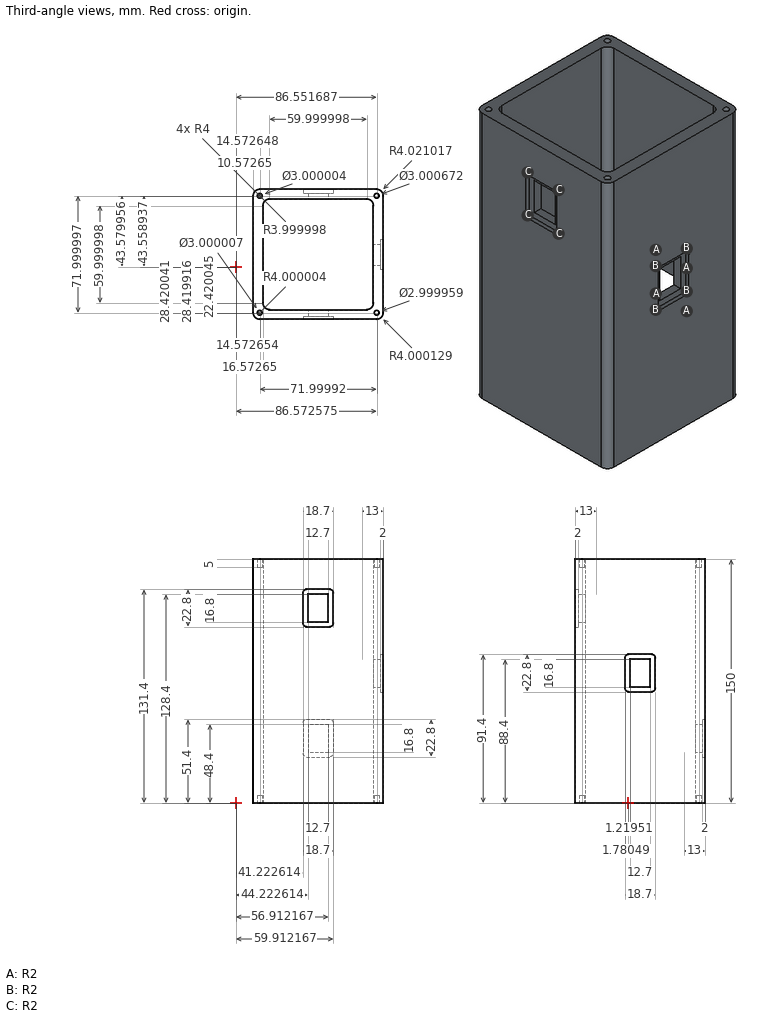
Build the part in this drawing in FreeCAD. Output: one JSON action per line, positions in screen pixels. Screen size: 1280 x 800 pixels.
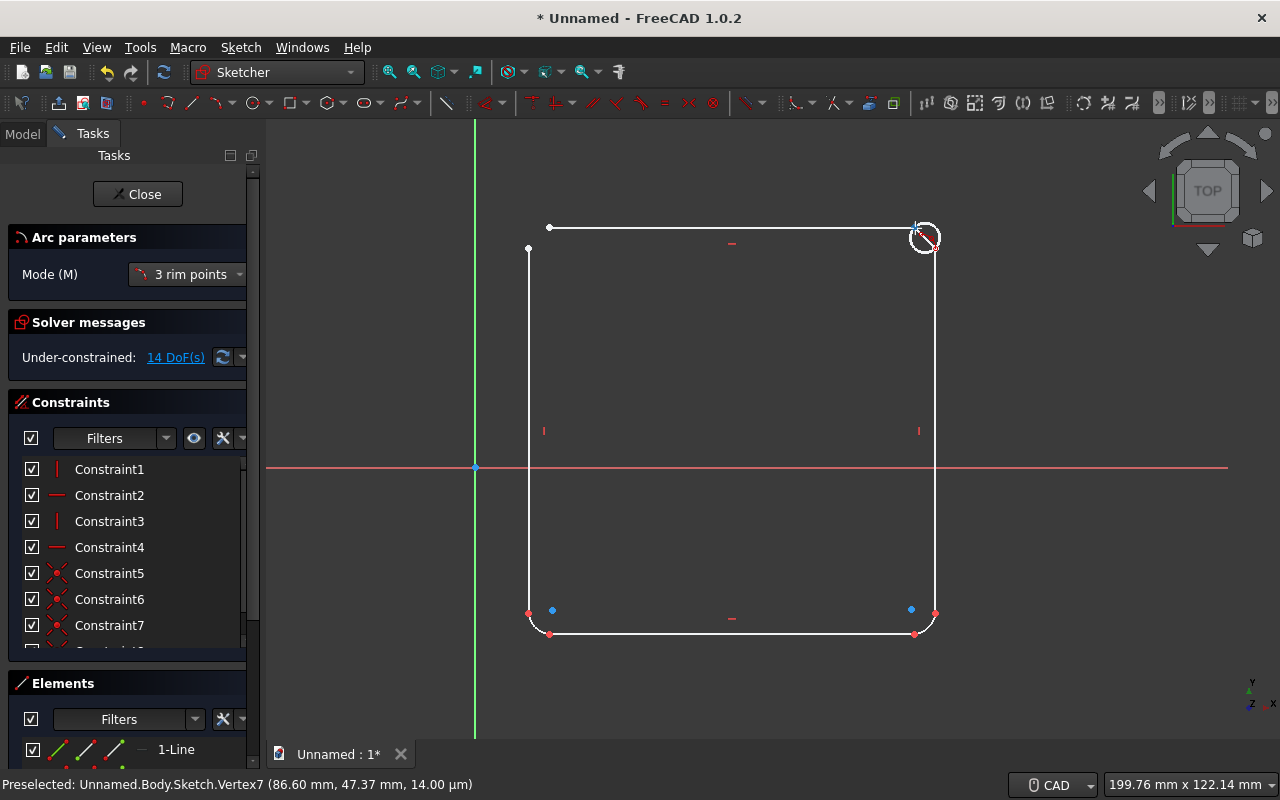
{"action": "scroll", "coordinate": [929, 232], "scroll_direction": "up", "scroll_amount": 5}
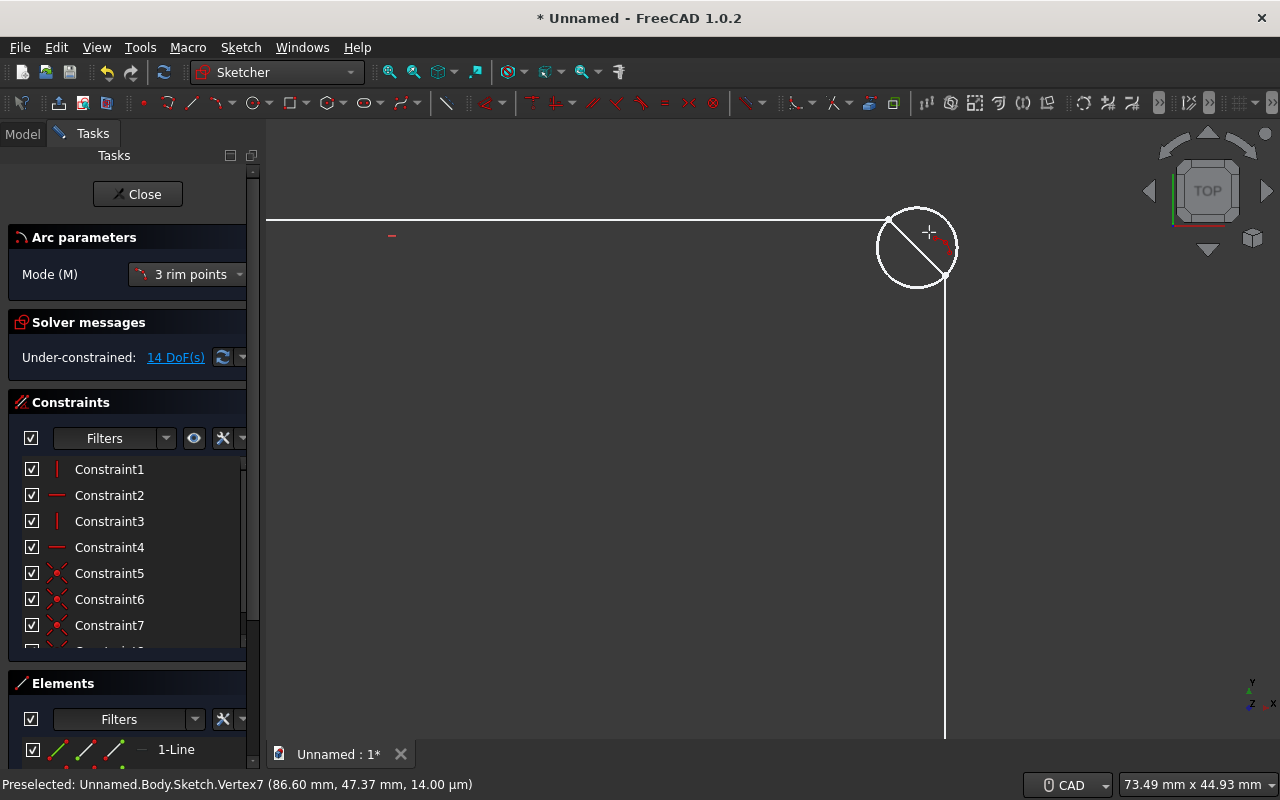
{"action": "left_click", "coordinate": [928, 233]}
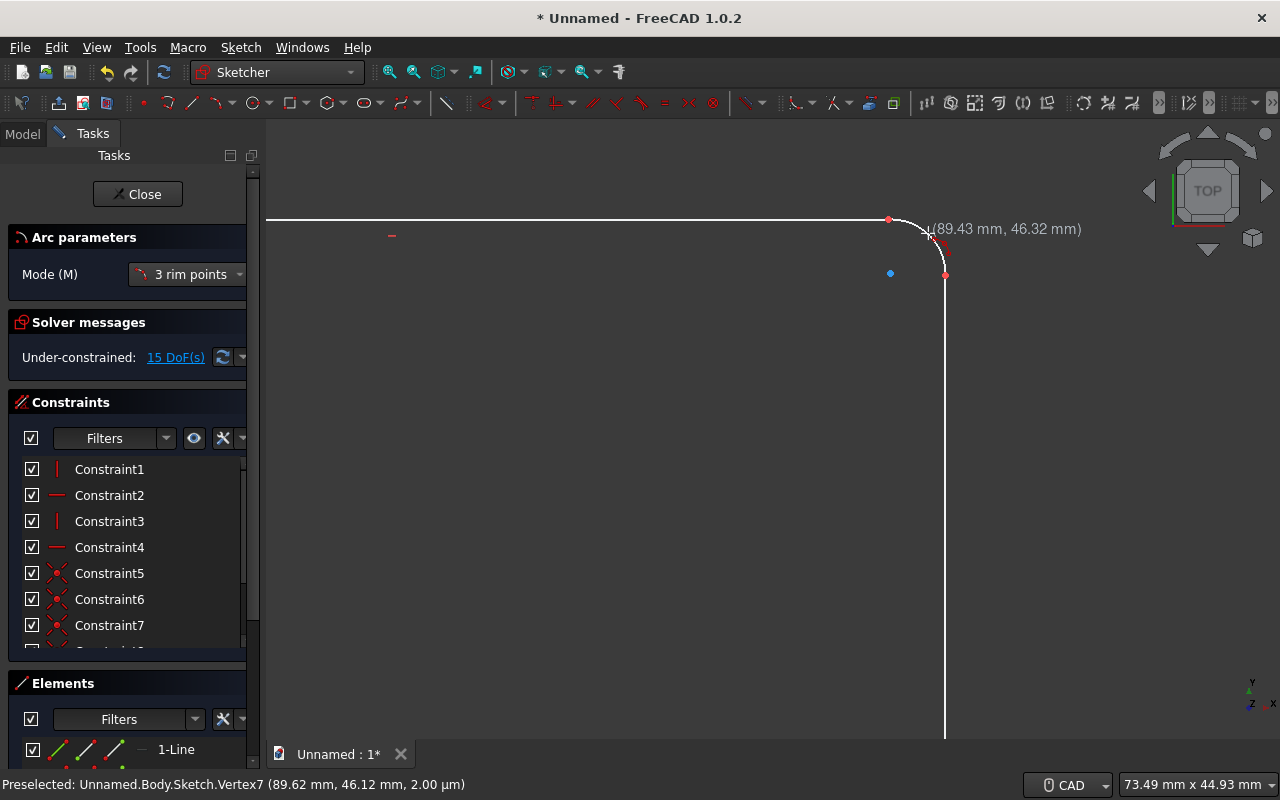
{"action": "scroll", "coordinate": [929, 231], "scroll_direction": "down", "scroll_amount": 5}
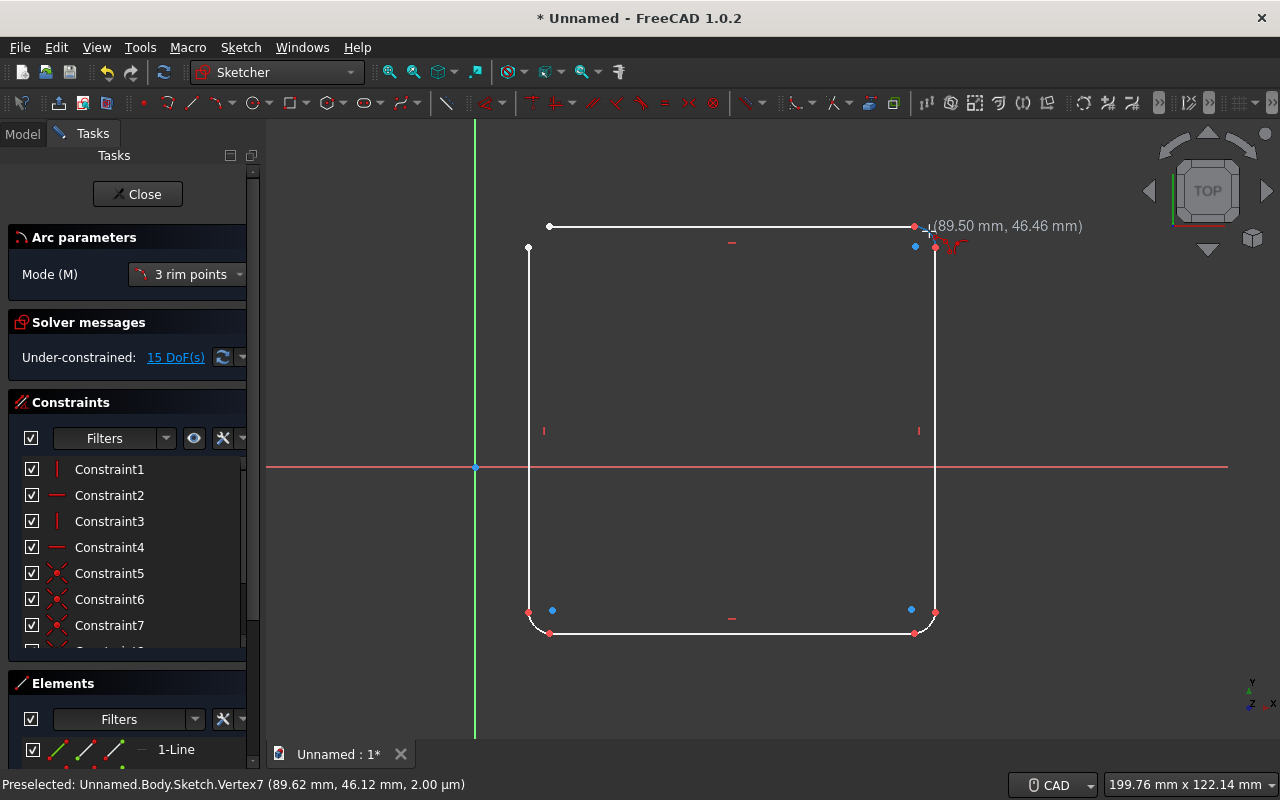
{"action": "left_click", "coordinate": [549, 227]}
{"action": "left_click", "coordinate": [529, 248]}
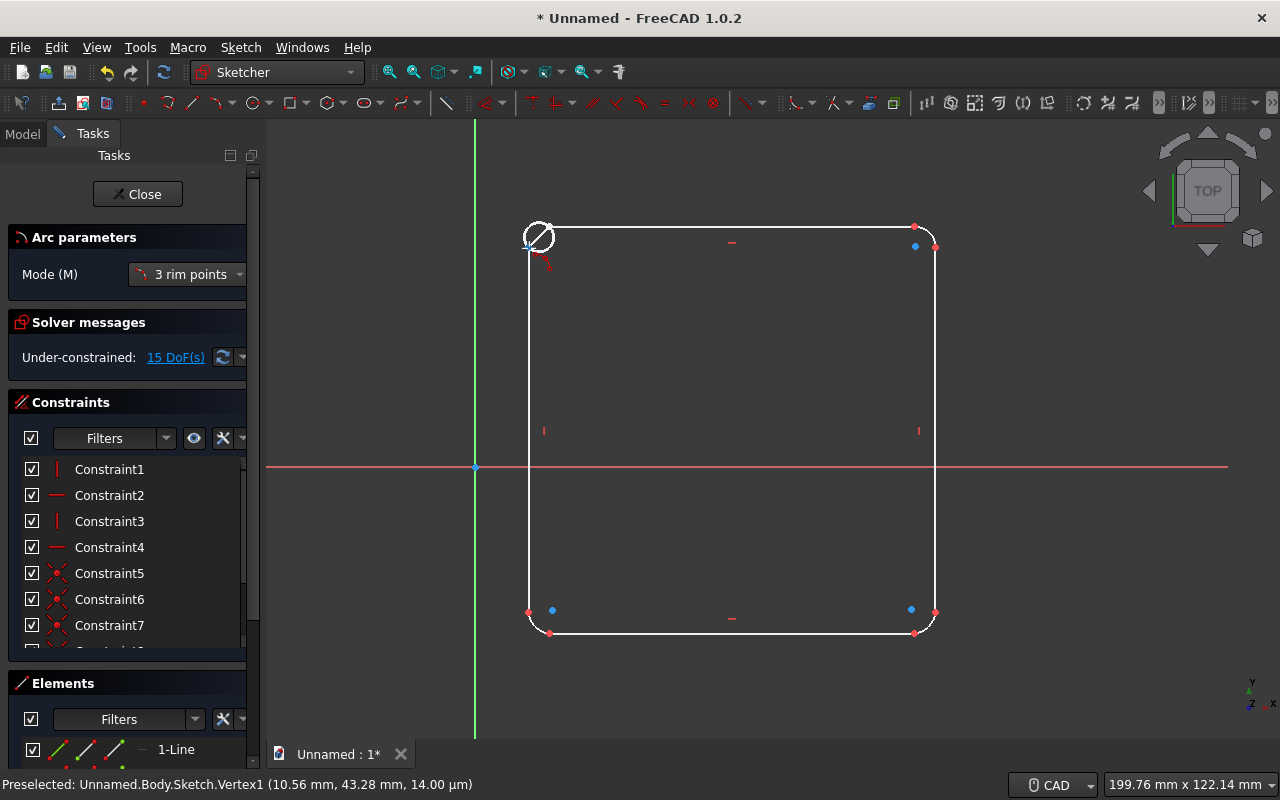
{"action": "scroll", "coordinate": [535, 232], "scroll_direction": "up", "scroll_amount": 5}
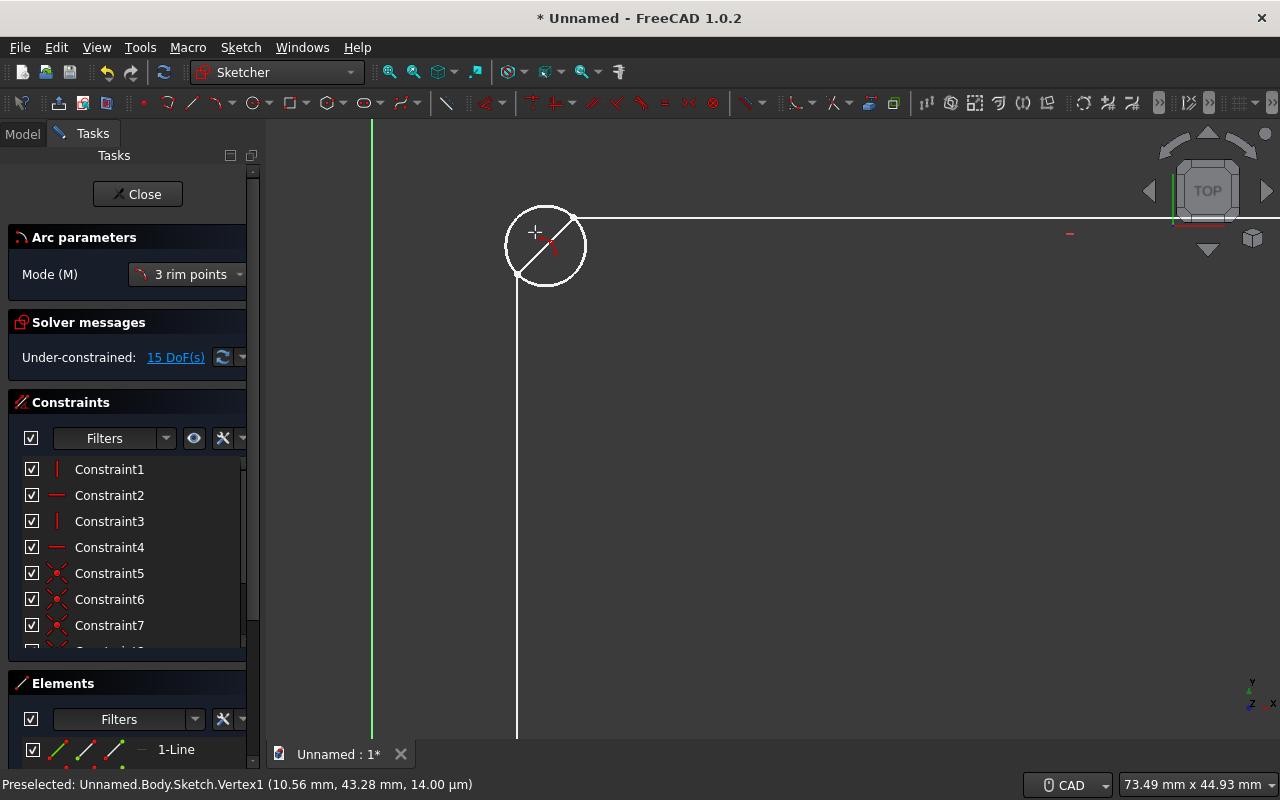
{"action": "left_click", "coordinate": [534, 231]}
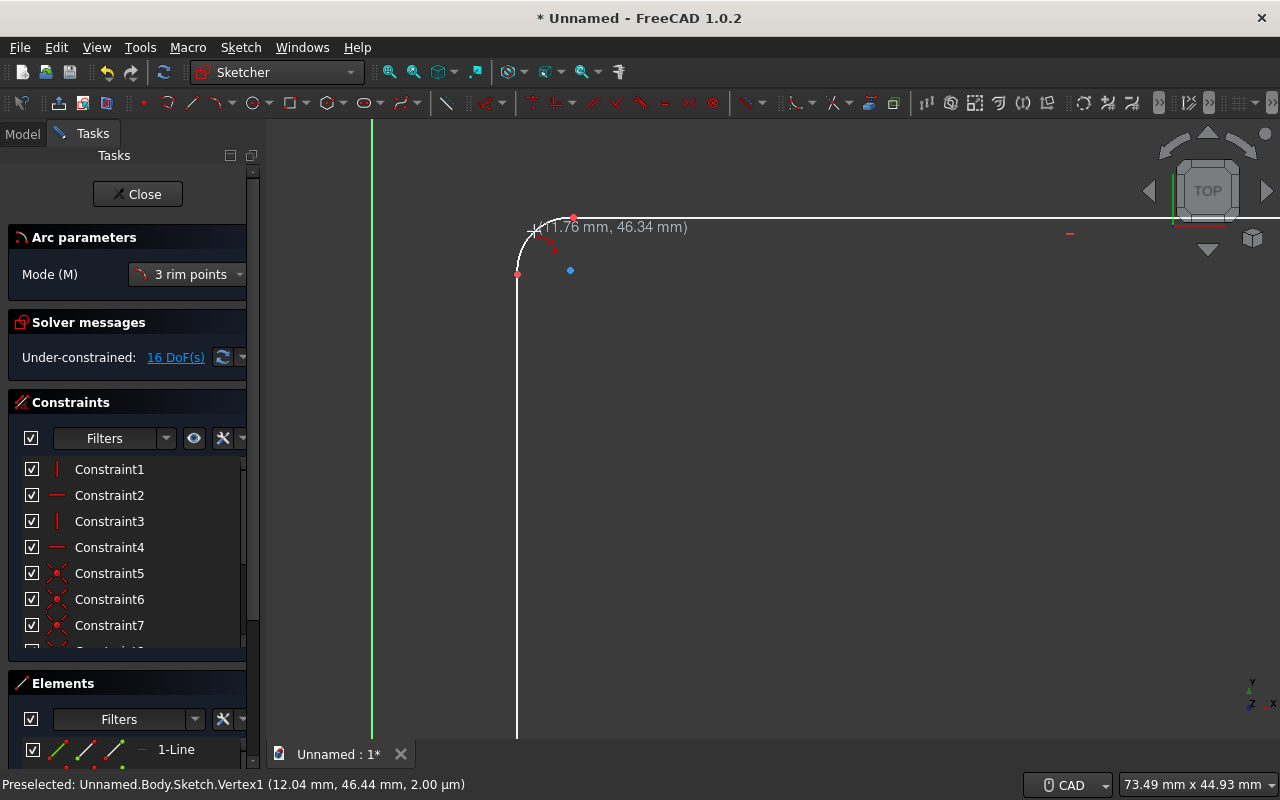
{"action": "key", "text": "g l"}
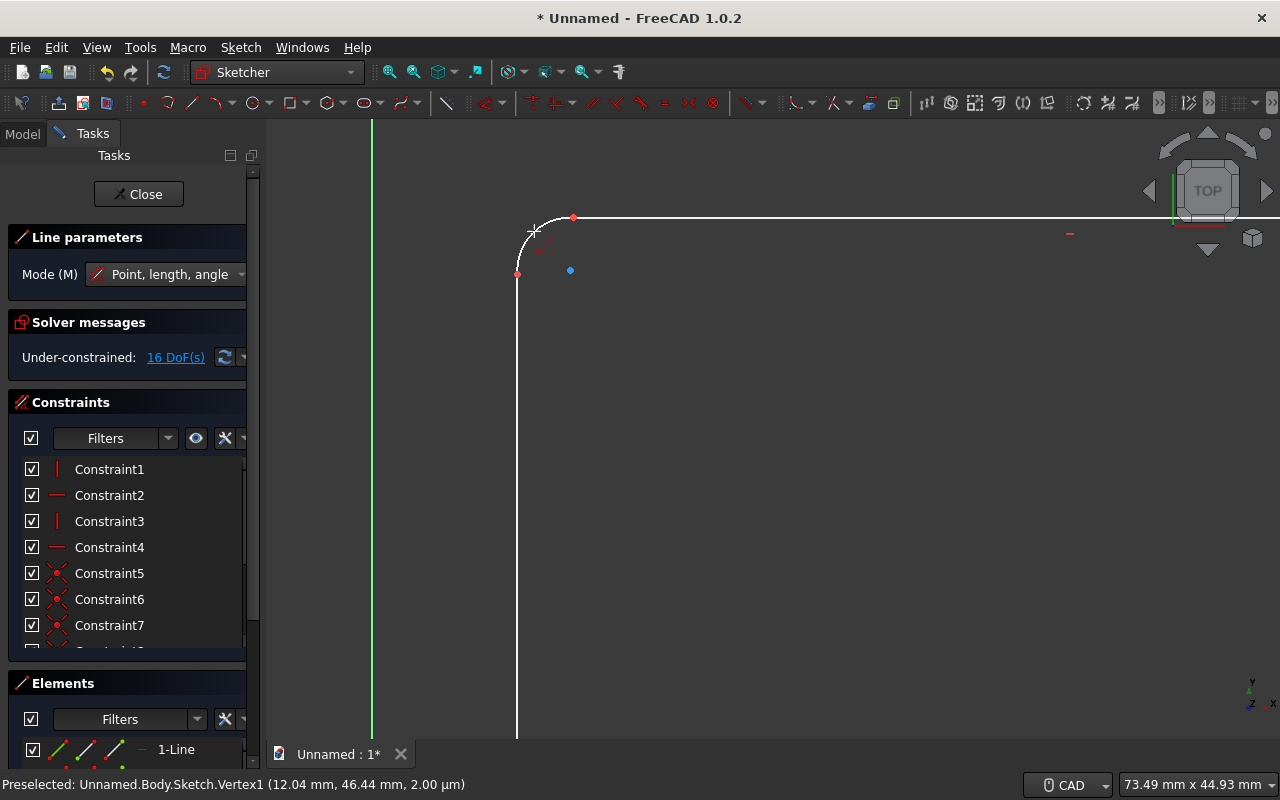
{"action": "scroll", "coordinate": [535, 232], "scroll_direction": "down", "scroll_amount": 5}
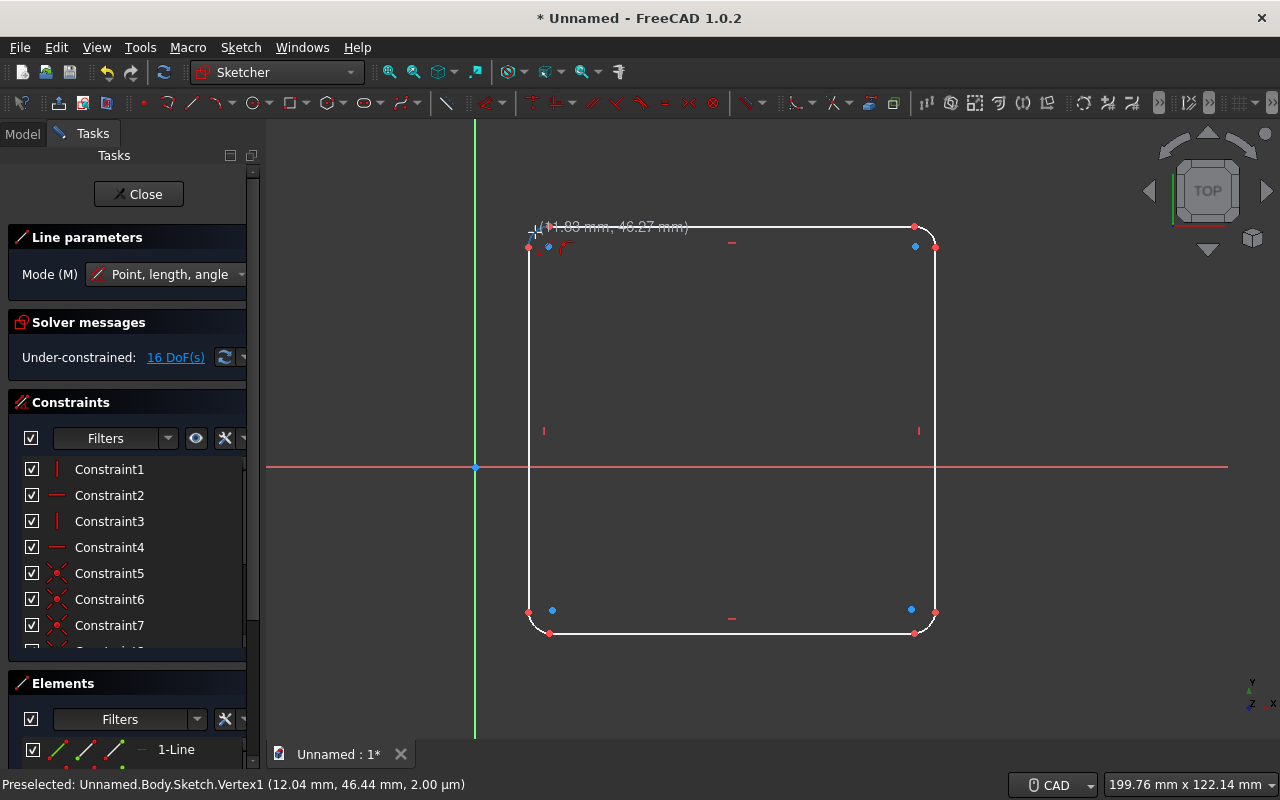
{"action": "left_click", "coordinate": [559, 581]}
{"action": "left_click", "coordinate": [559, 277]}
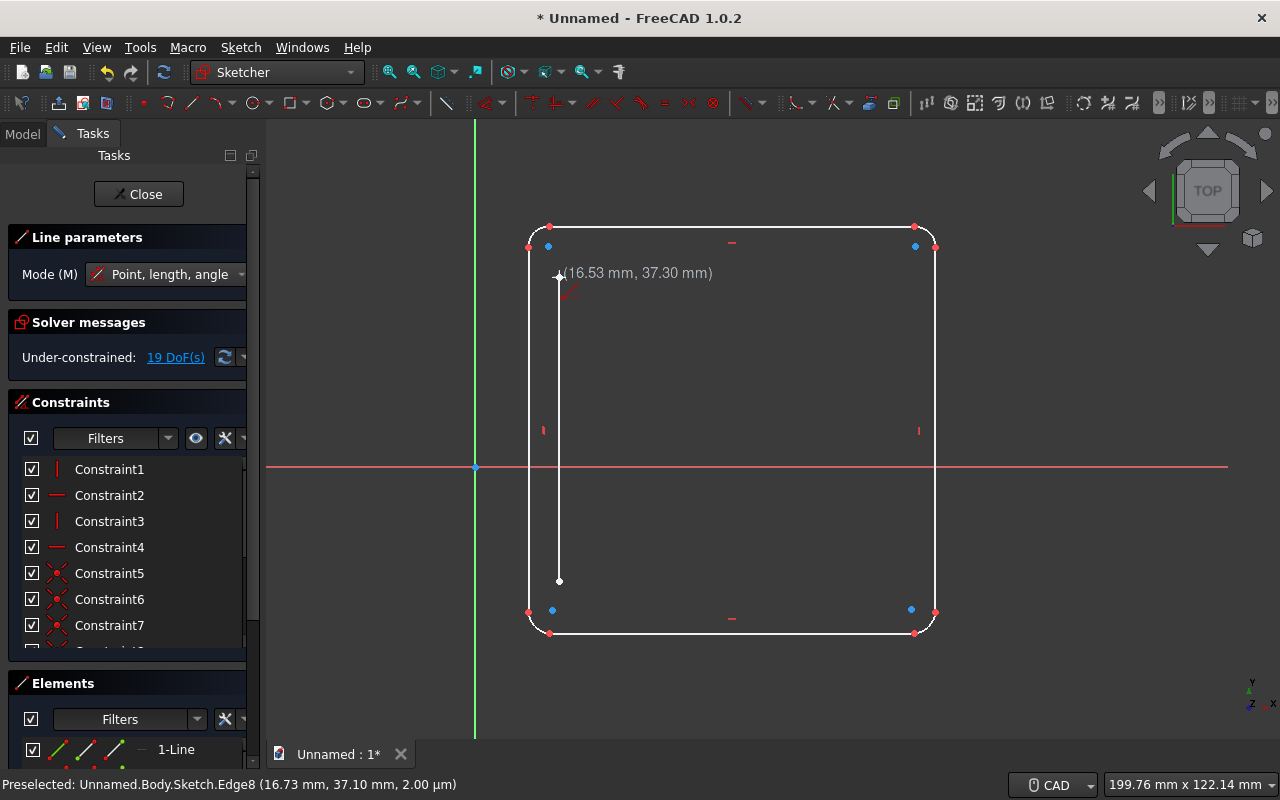
{"action": "left_click", "coordinate": [580, 256]}
{"action": "left_click", "coordinate": [884, 256]}